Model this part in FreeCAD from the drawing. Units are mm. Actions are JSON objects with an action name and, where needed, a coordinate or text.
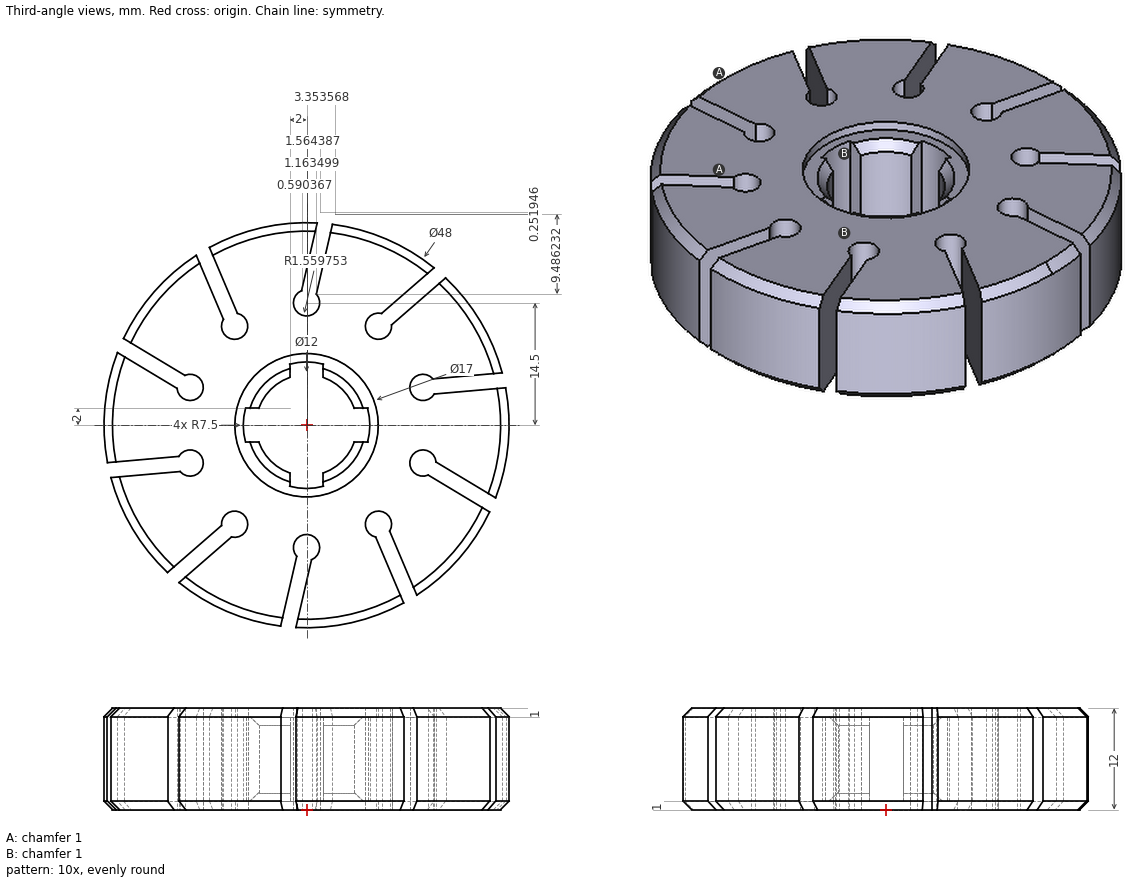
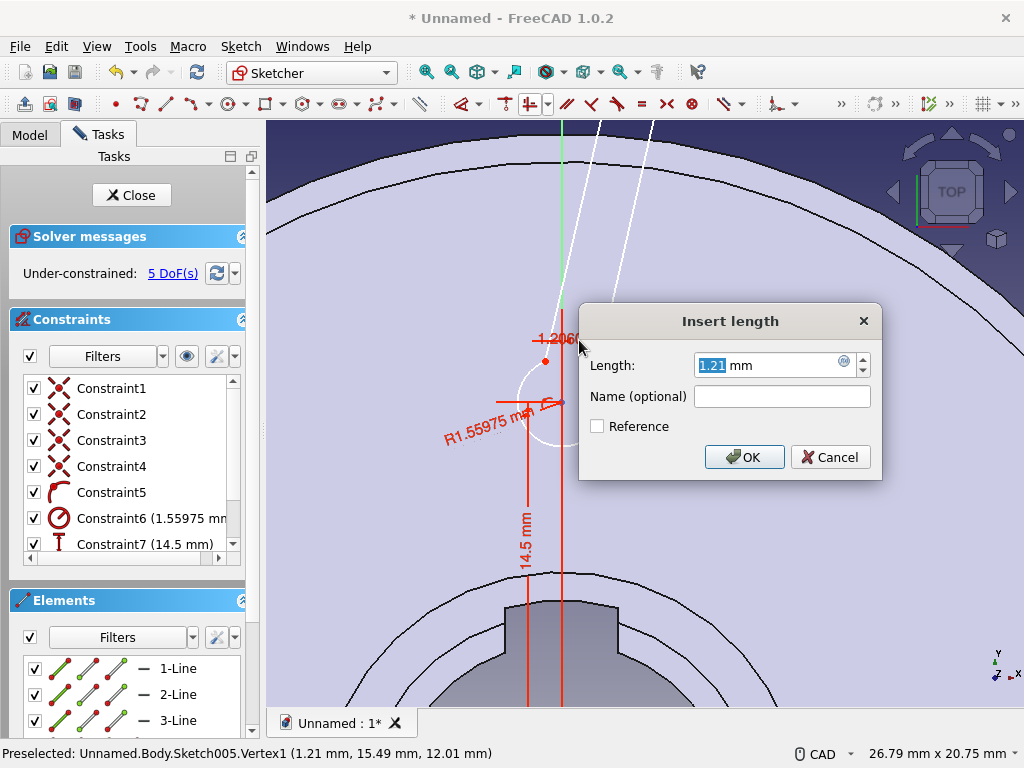
{"action": "type", "text": "1.163499"}
{"action": "key", "text": "Return"}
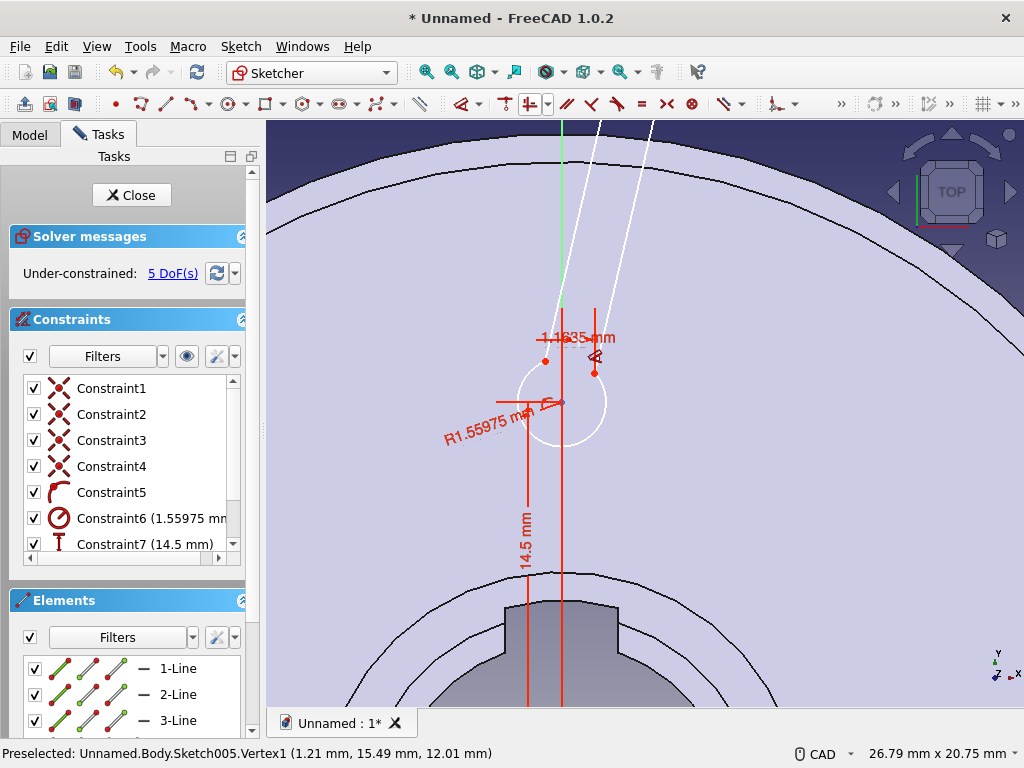
{"action": "scroll", "coordinate": [547, 363], "scroll_direction": "down", "scroll_amount": 3}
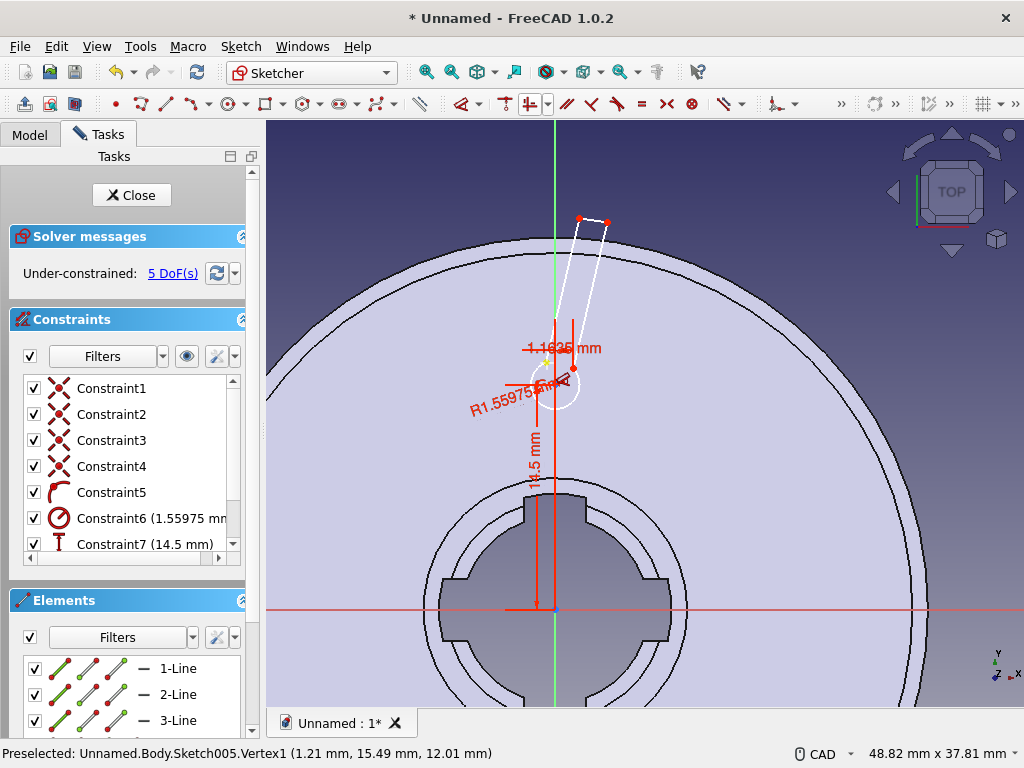
{"action": "left_click", "coordinate": [607, 222]}
{"action": "left_click", "coordinate": [581, 644]}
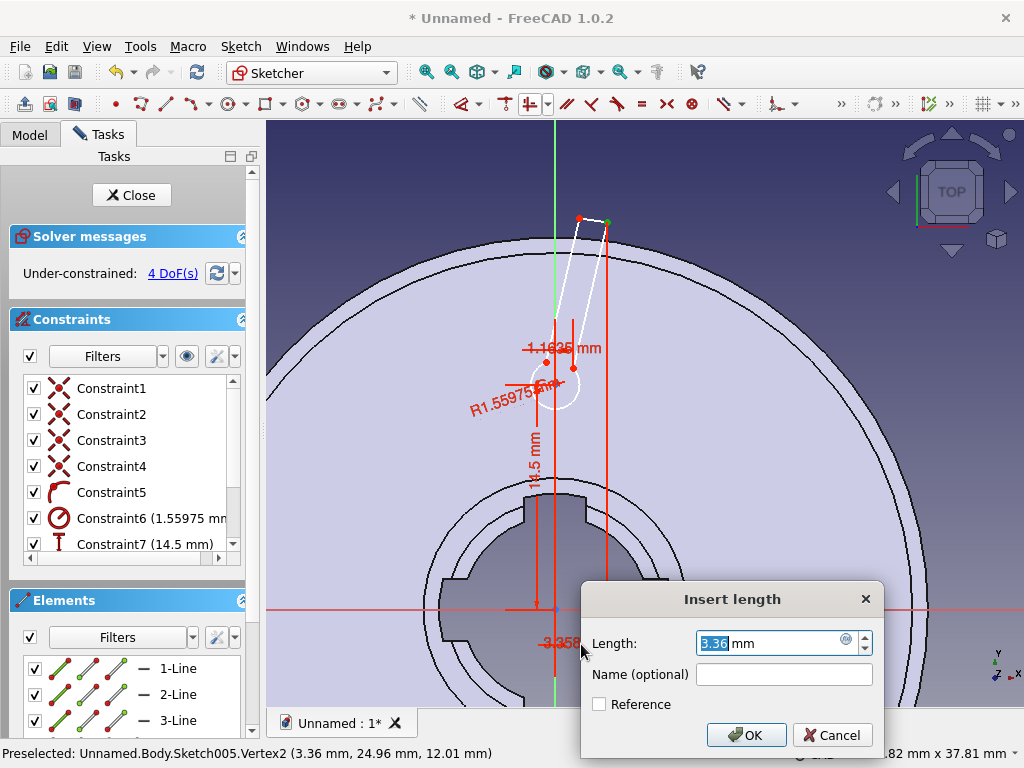
{"action": "type", "text": "3.353568"}
{"action": "key", "text": "Return"}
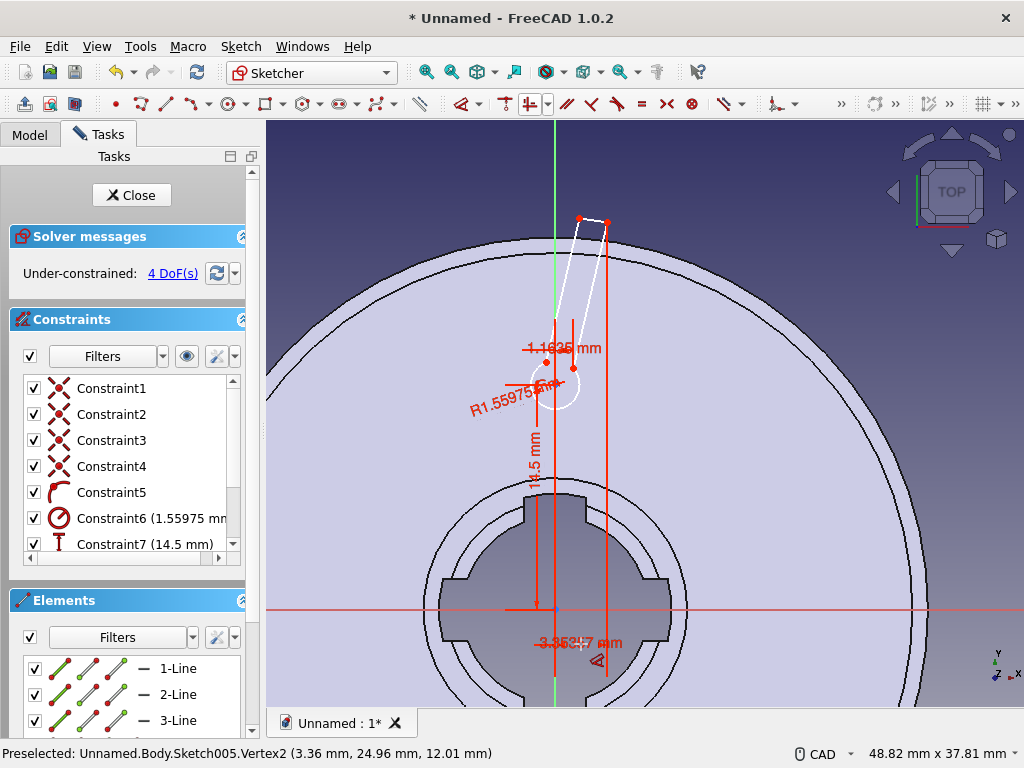
{"action": "scroll", "coordinate": [579, 218], "scroll_direction": "up", "scroll_amount": 3}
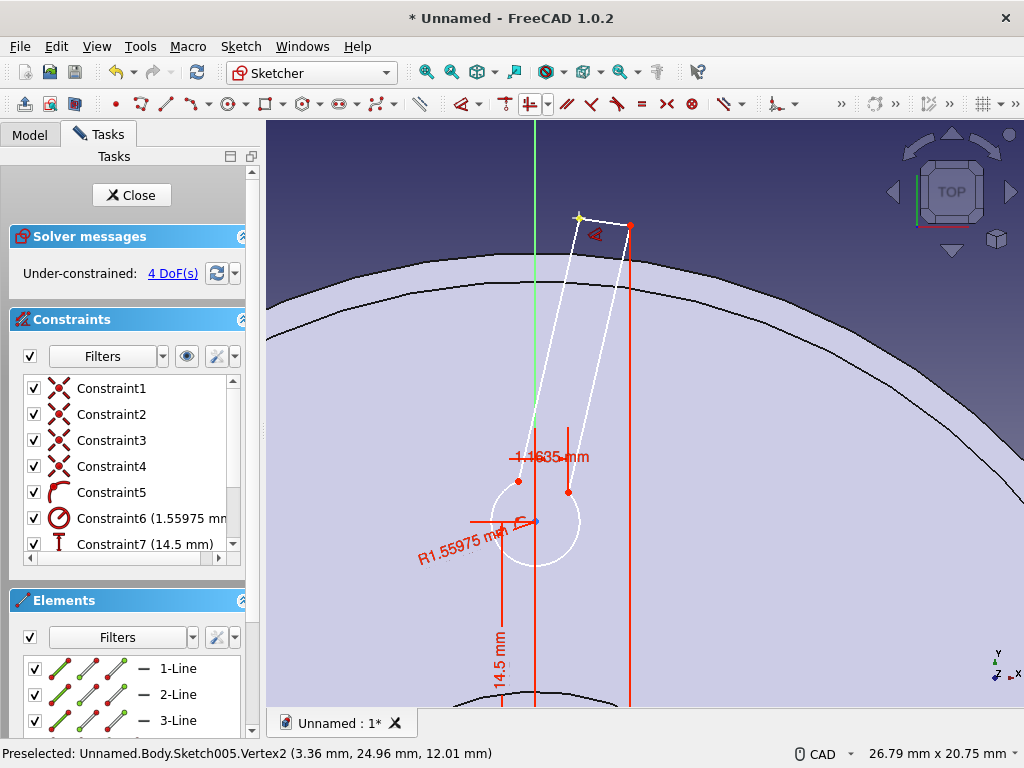
{"action": "left_click", "coordinate": [579, 219]}
{"action": "left_click", "coordinate": [557, 185]}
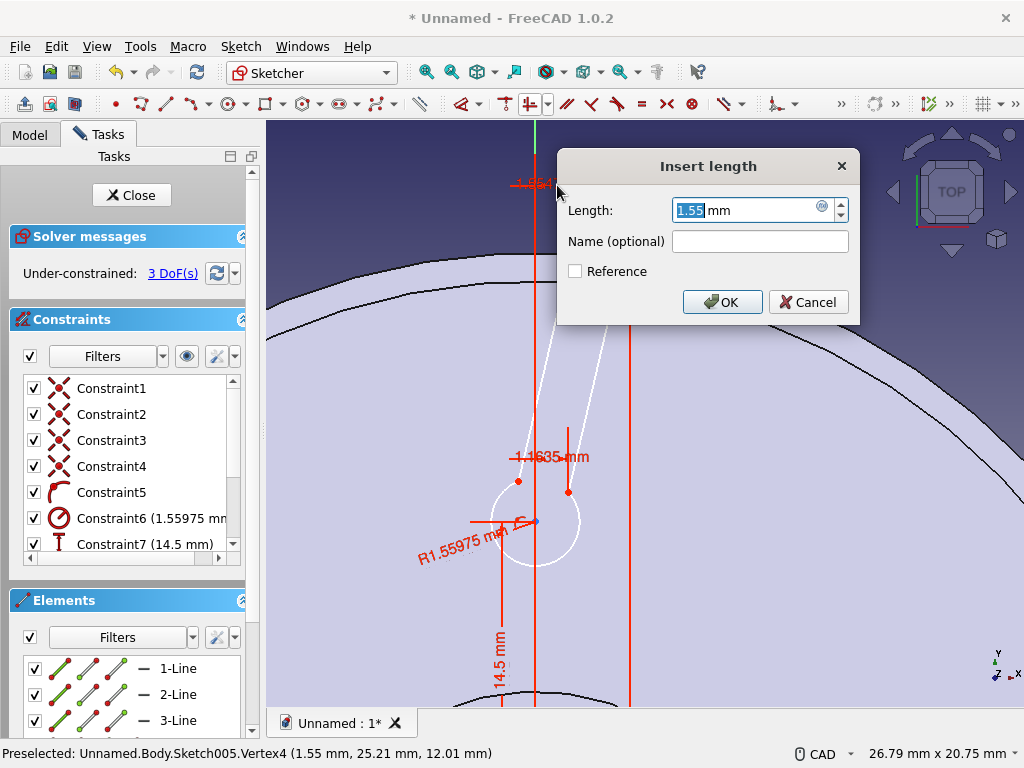
{"action": "type", "text": "1.564387"}
{"action": "key", "text": "Return"}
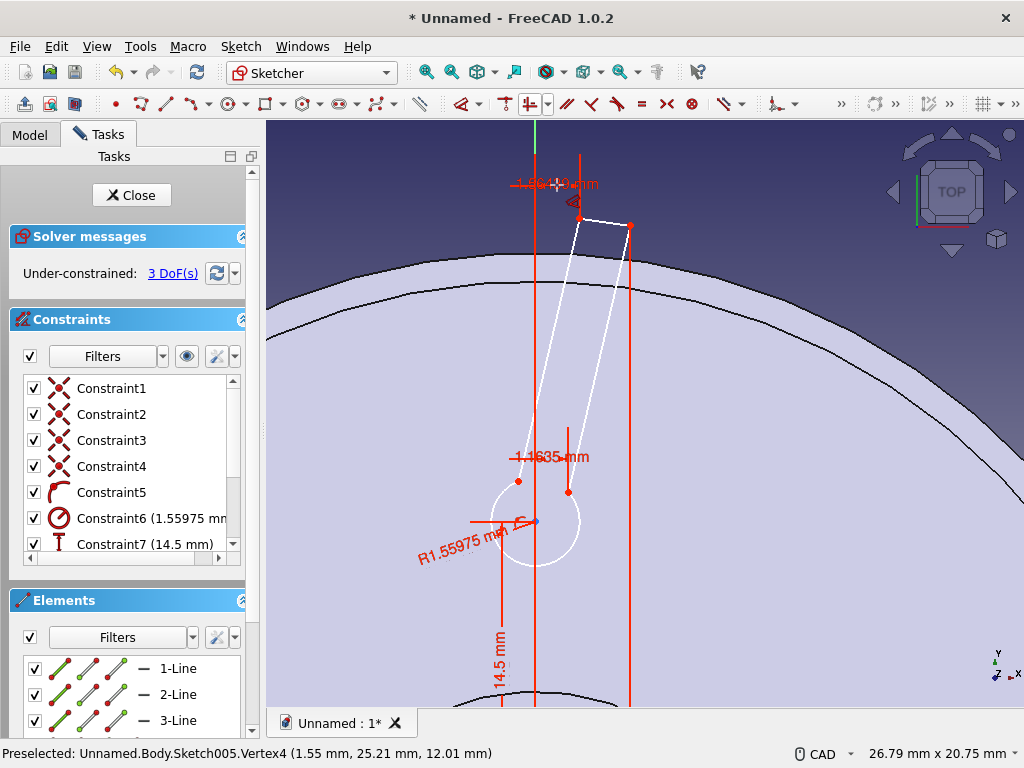
{"action": "scroll", "coordinate": [519, 481], "scroll_direction": "up", "scroll_amount": 5}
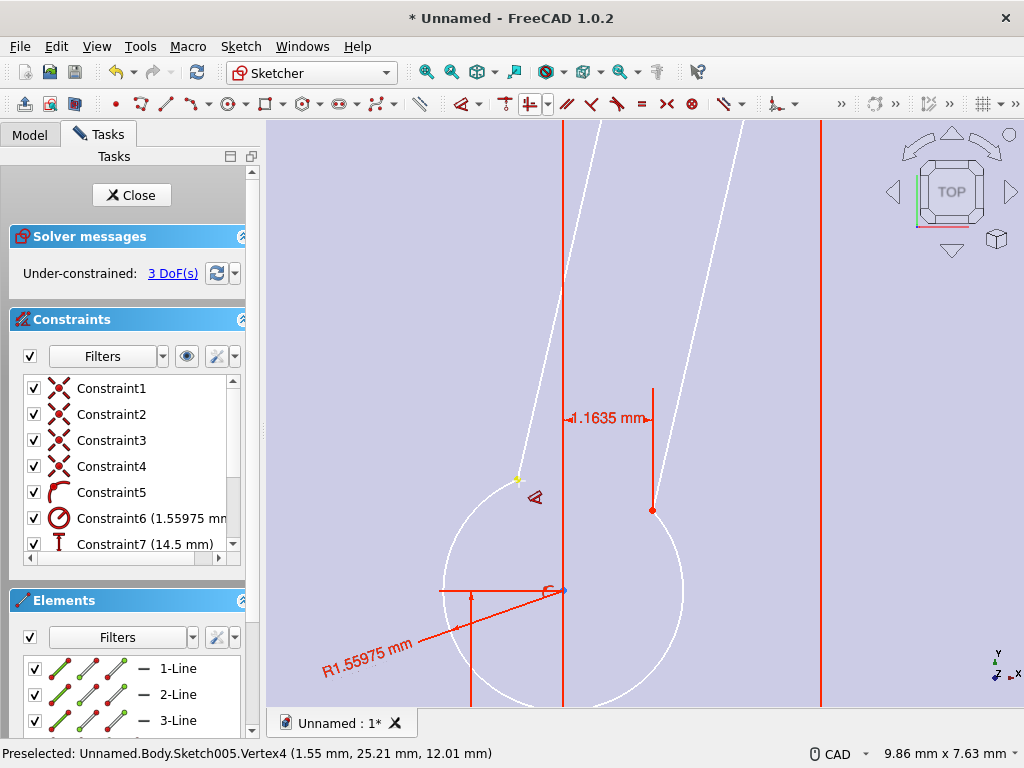
{"action": "left_click", "coordinate": [517, 480]}
{"action": "left_click", "coordinate": [540, 446]}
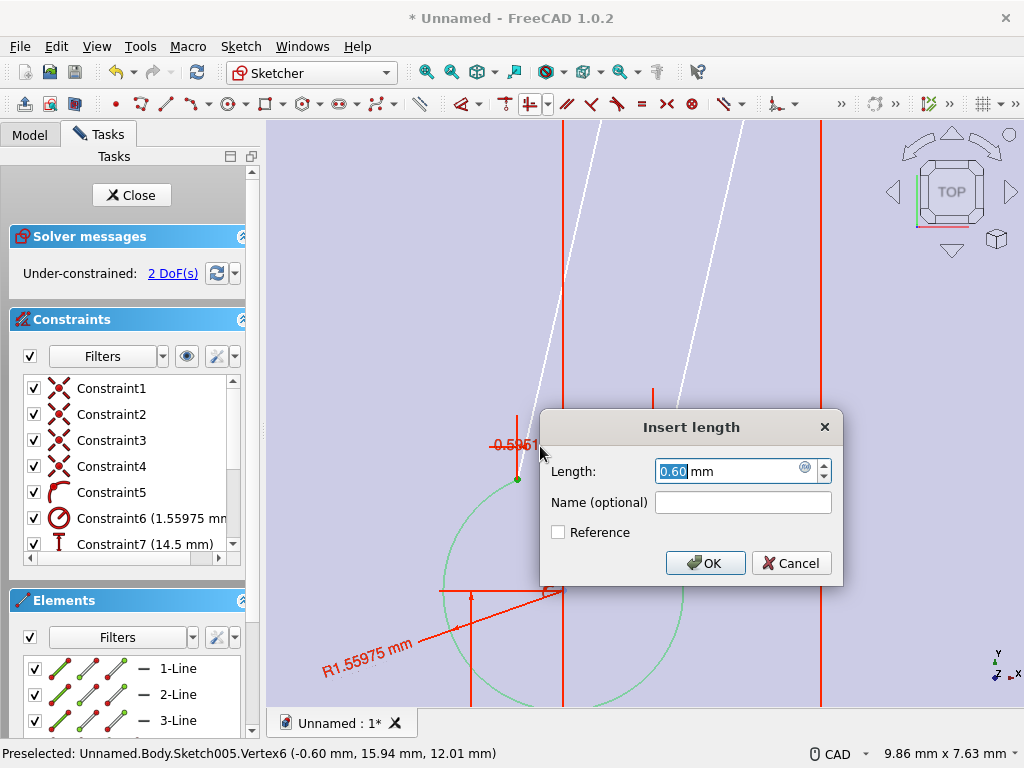
{"action": "type", "text": "0.590367"}
{"action": "key", "text": "Return"}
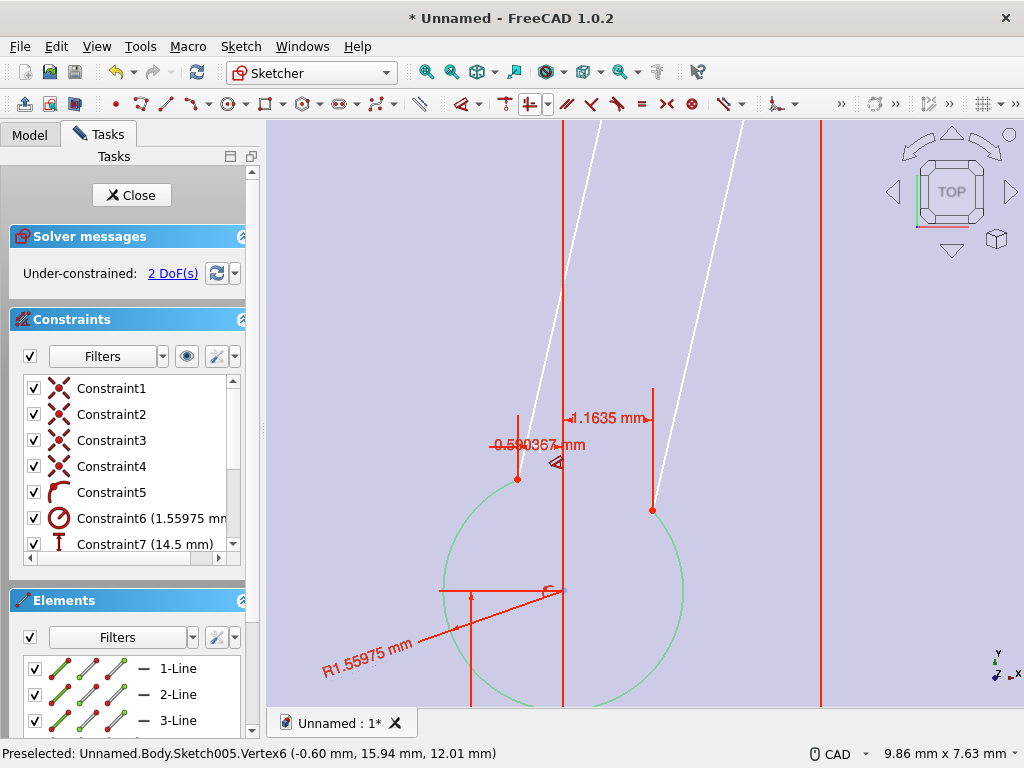
{"action": "scroll", "coordinate": [553, 332], "scroll_direction": "down", "scroll_amount": 8}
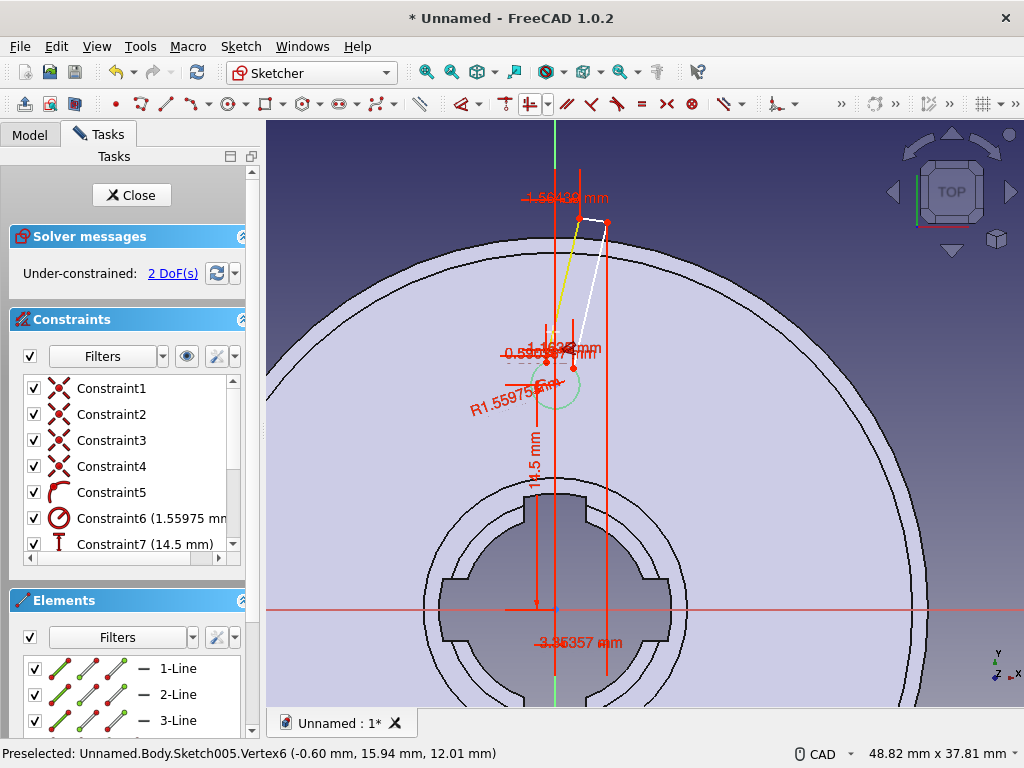
{"action": "left_click", "coordinate": [584, 325]}
{"action": "left_click", "coordinate": [641, 295]}